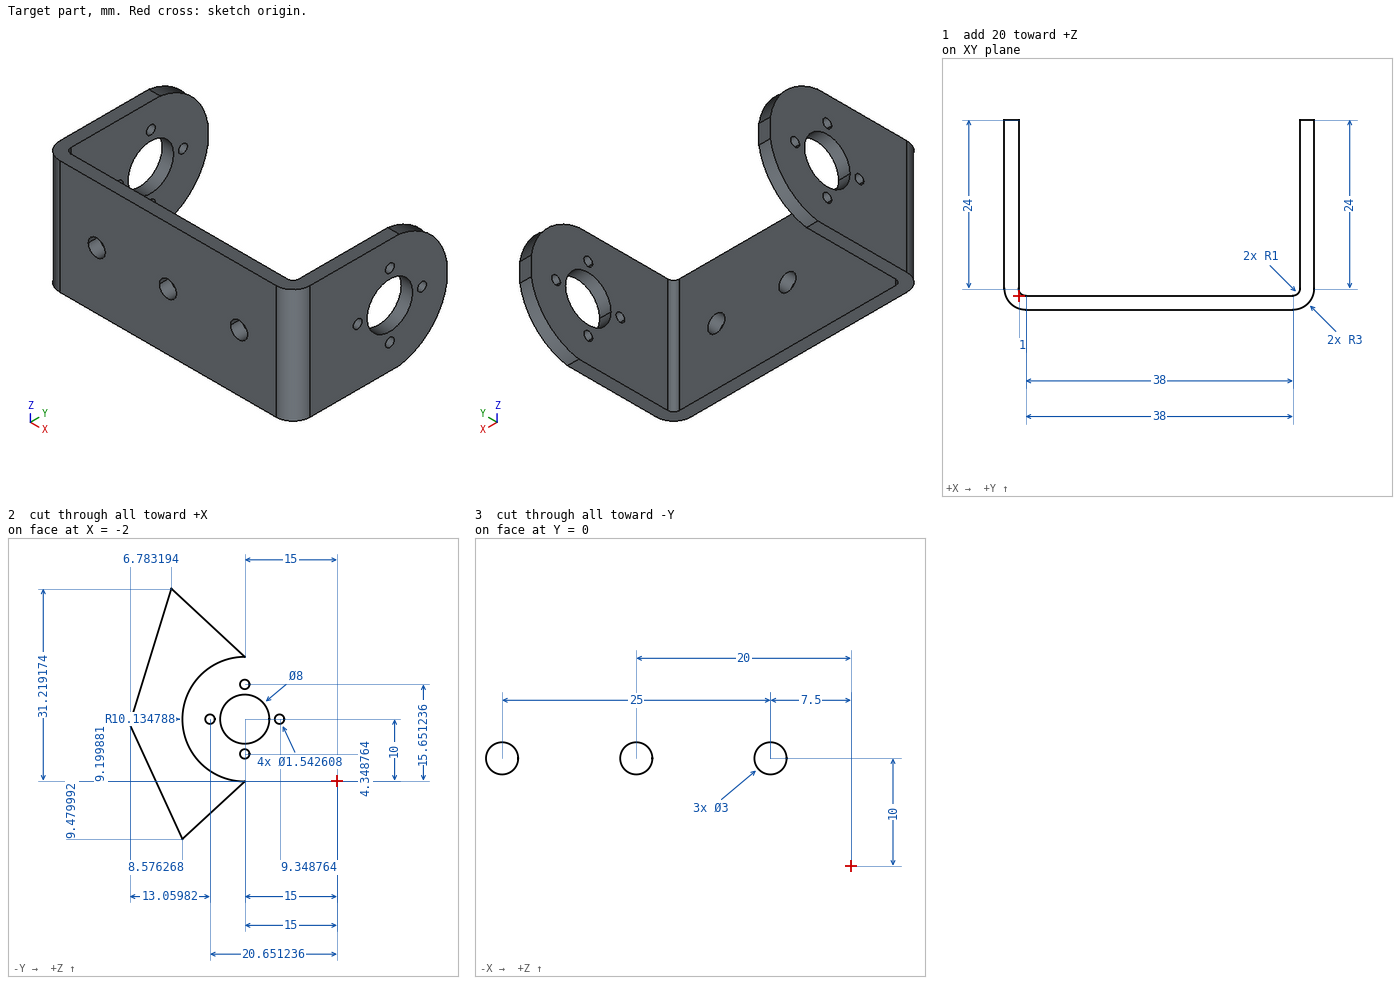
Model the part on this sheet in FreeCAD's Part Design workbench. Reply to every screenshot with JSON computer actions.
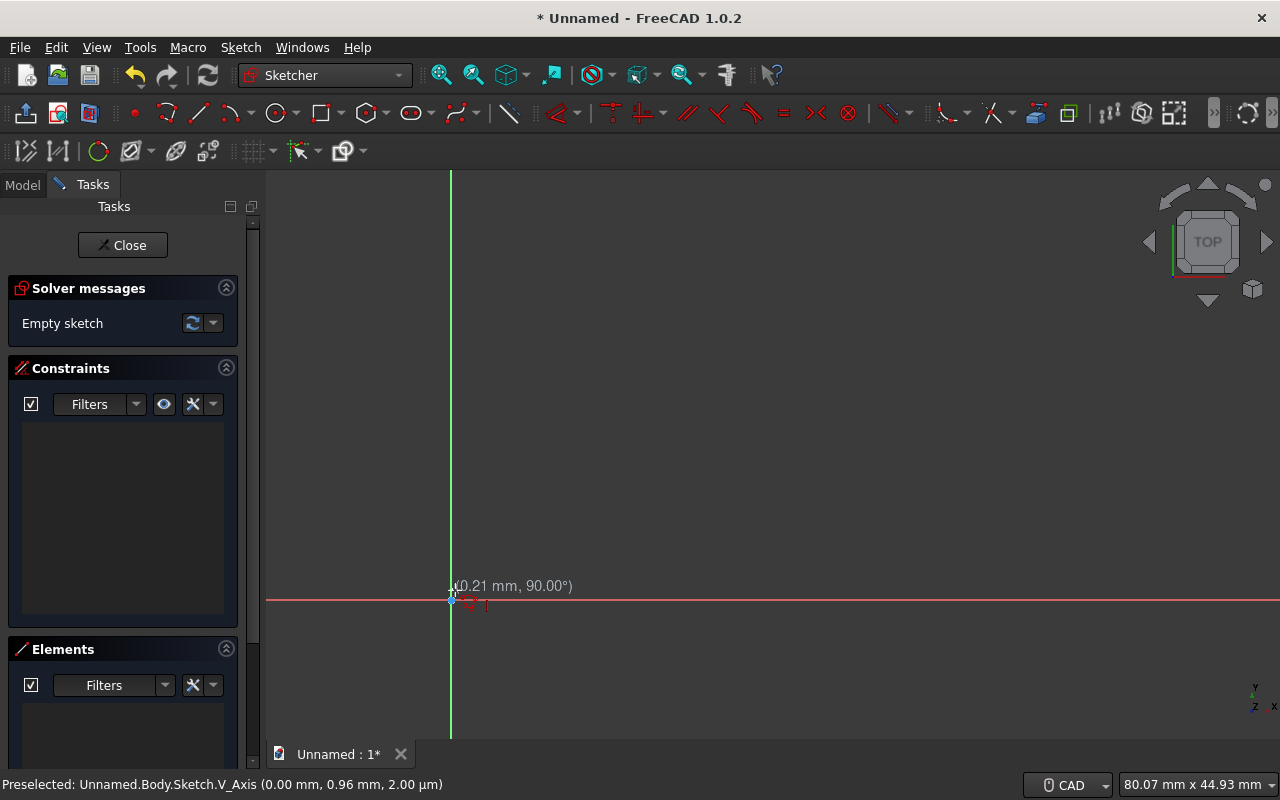
{"action": "left_click", "coordinate": [460, 284]}
{"action": "left_click", "coordinate": [426, 284]}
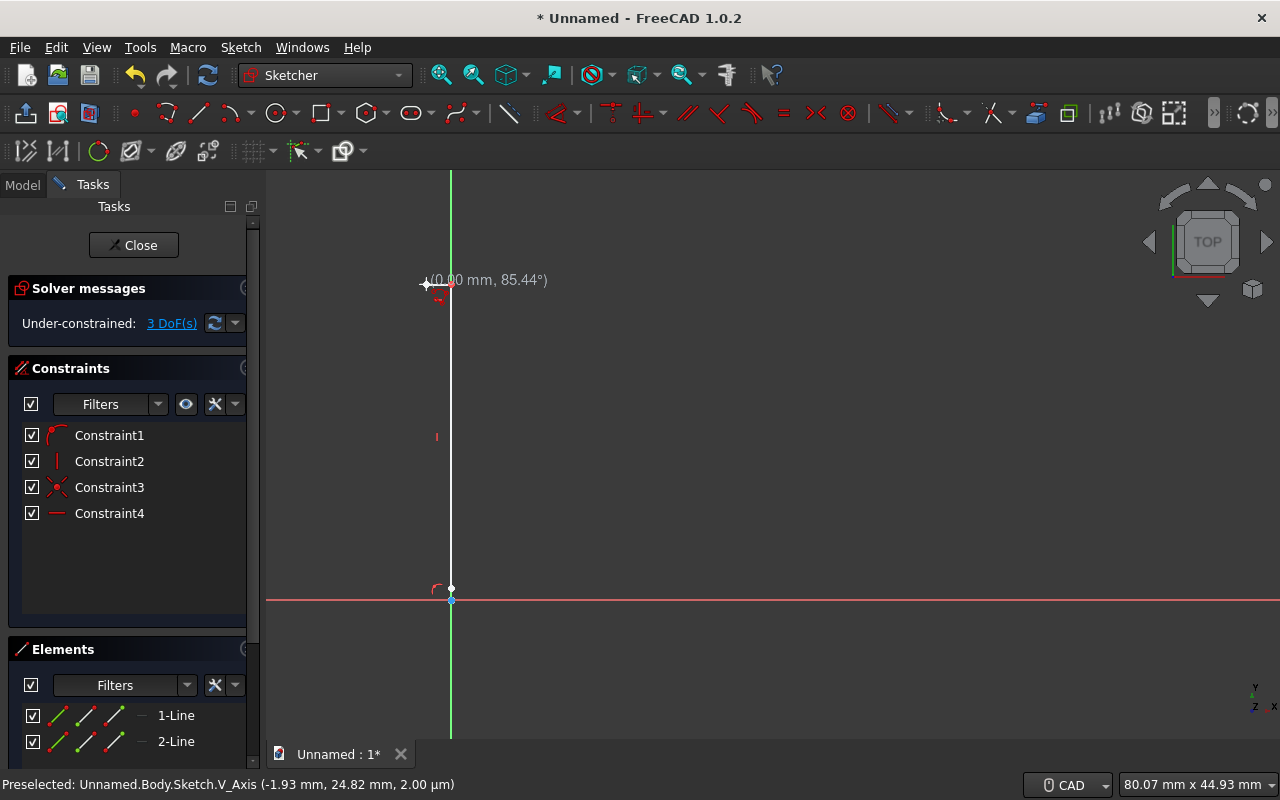
{"action": "scroll", "coordinate": [426, 588], "scroll_direction": "up", "scroll_amount": 2}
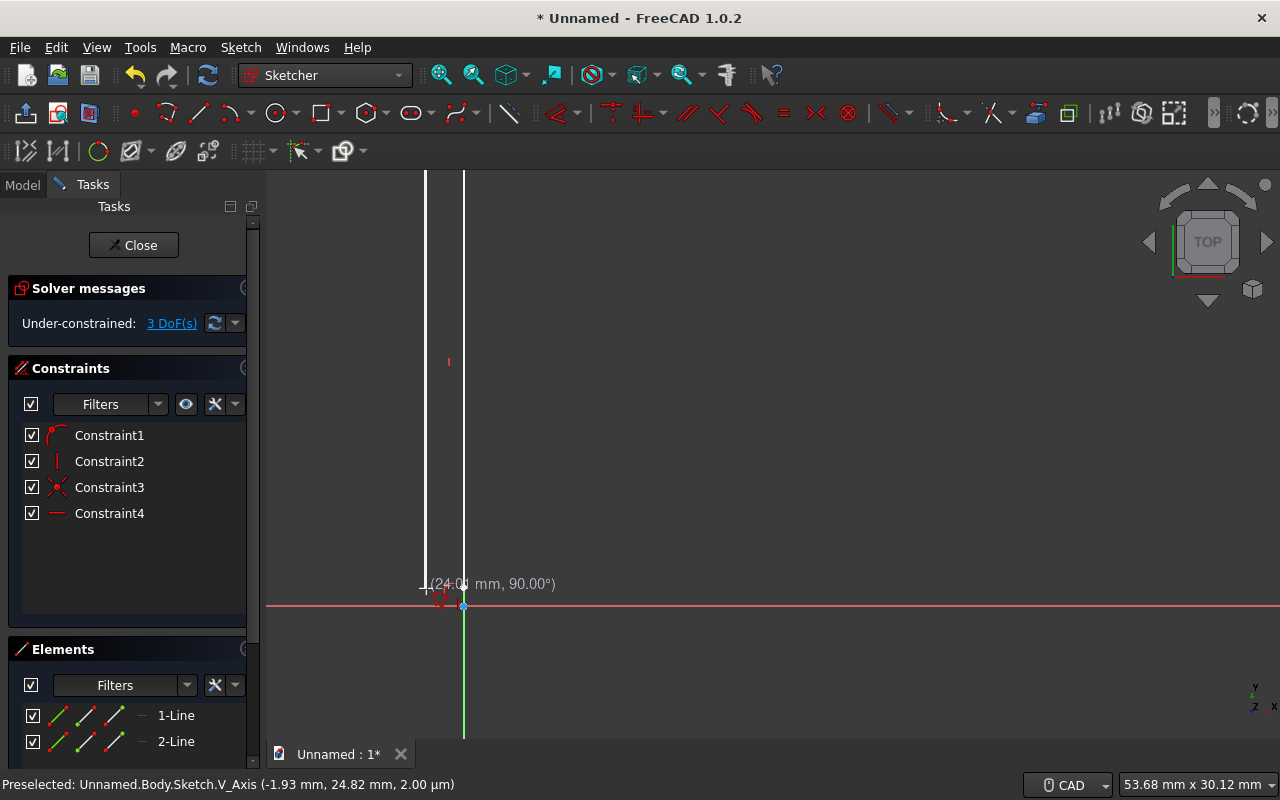
{"action": "left_click", "coordinate": [426, 587]}
{"action": "right_click", "coordinate": [426, 587]}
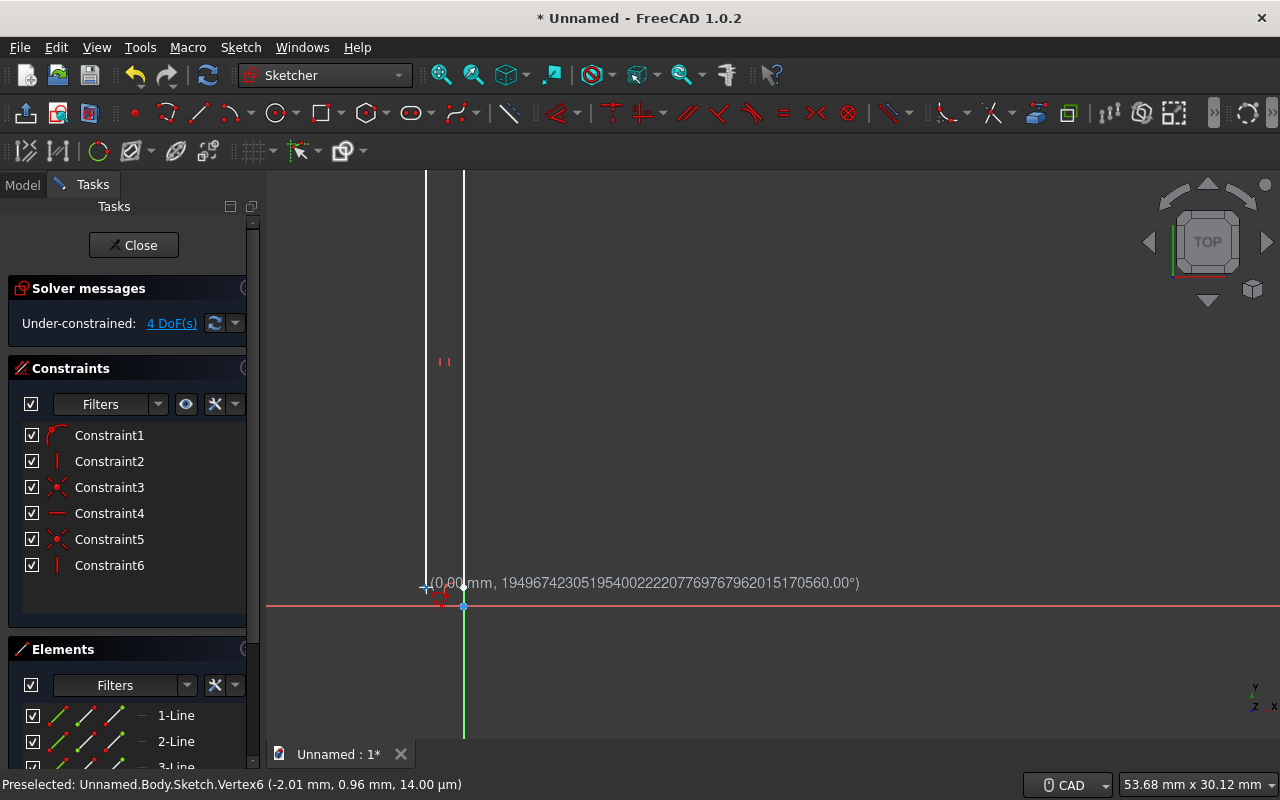
{"action": "left_click", "coordinate": [200, 114]}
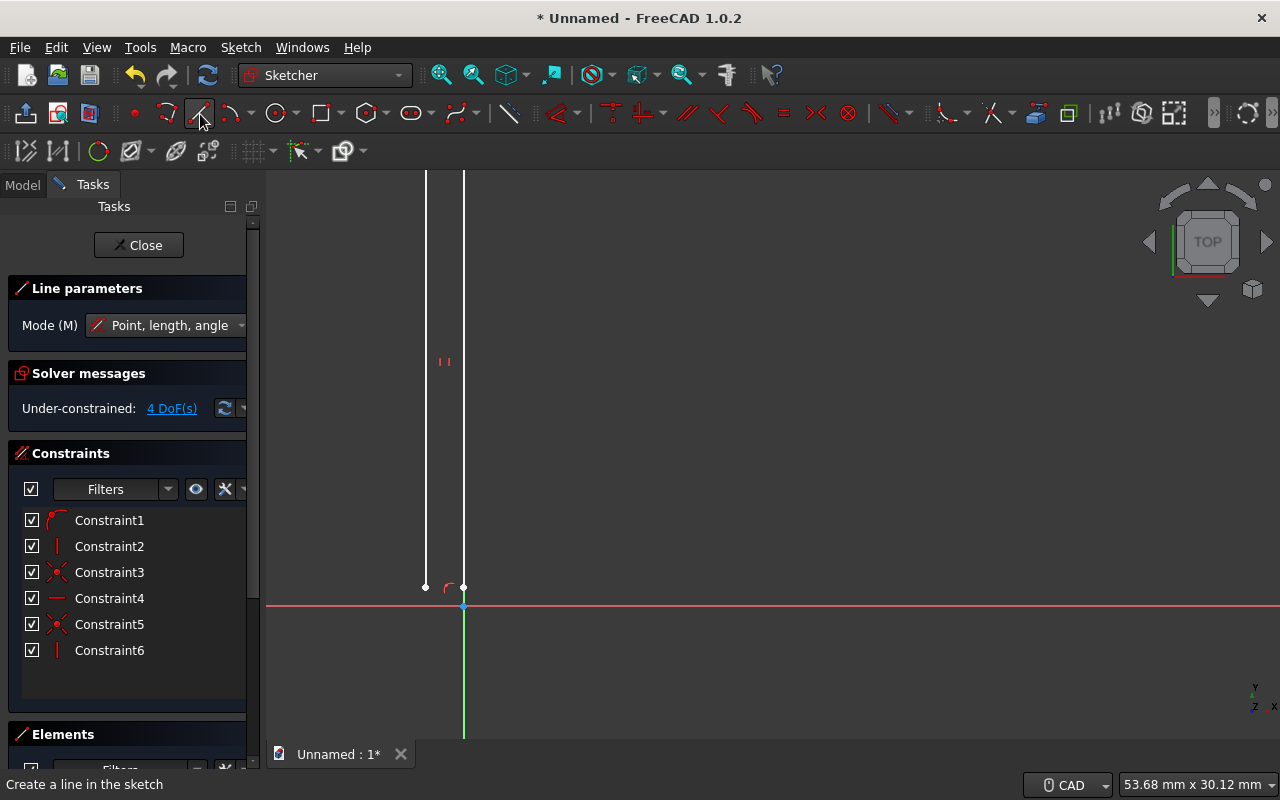
{"action": "left_click", "coordinate": [483, 644]}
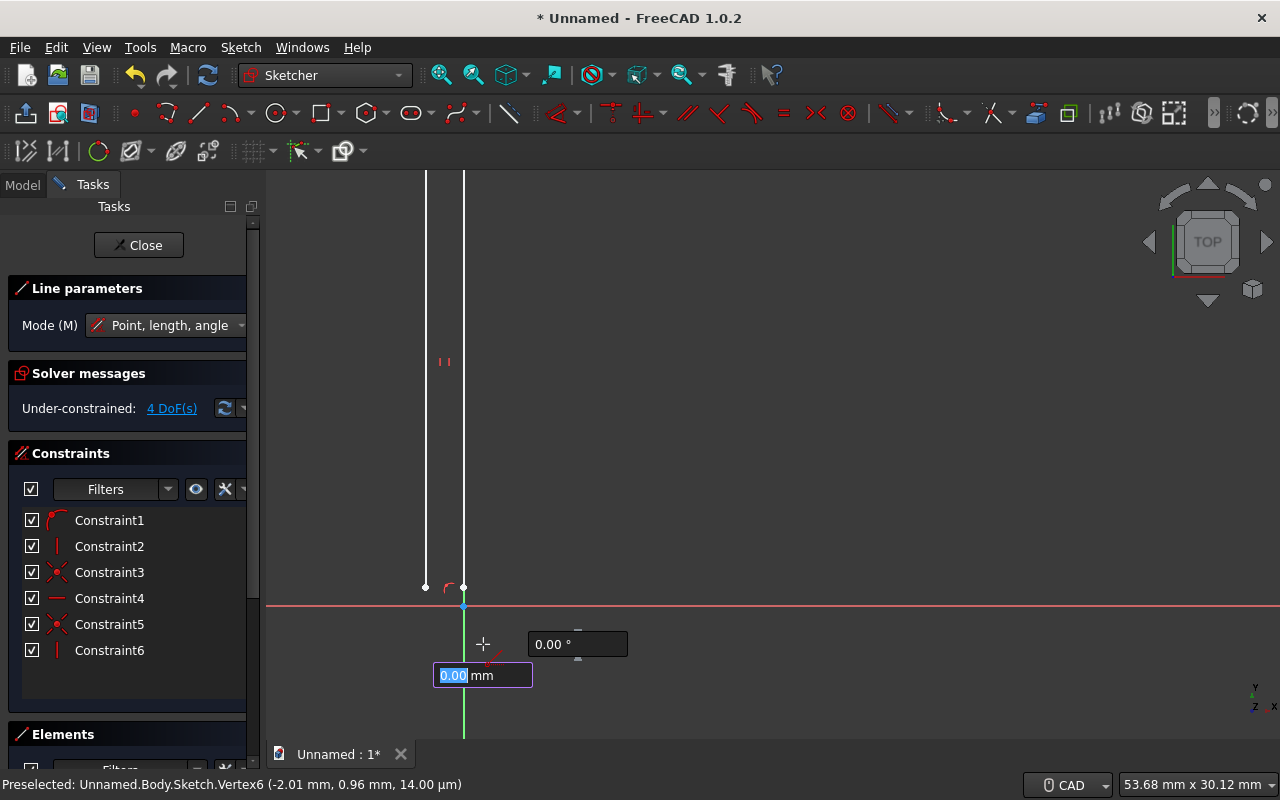
{"action": "scroll", "coordinate": [426, 588], "scroll_direction": "down", "scroll_amount": 2}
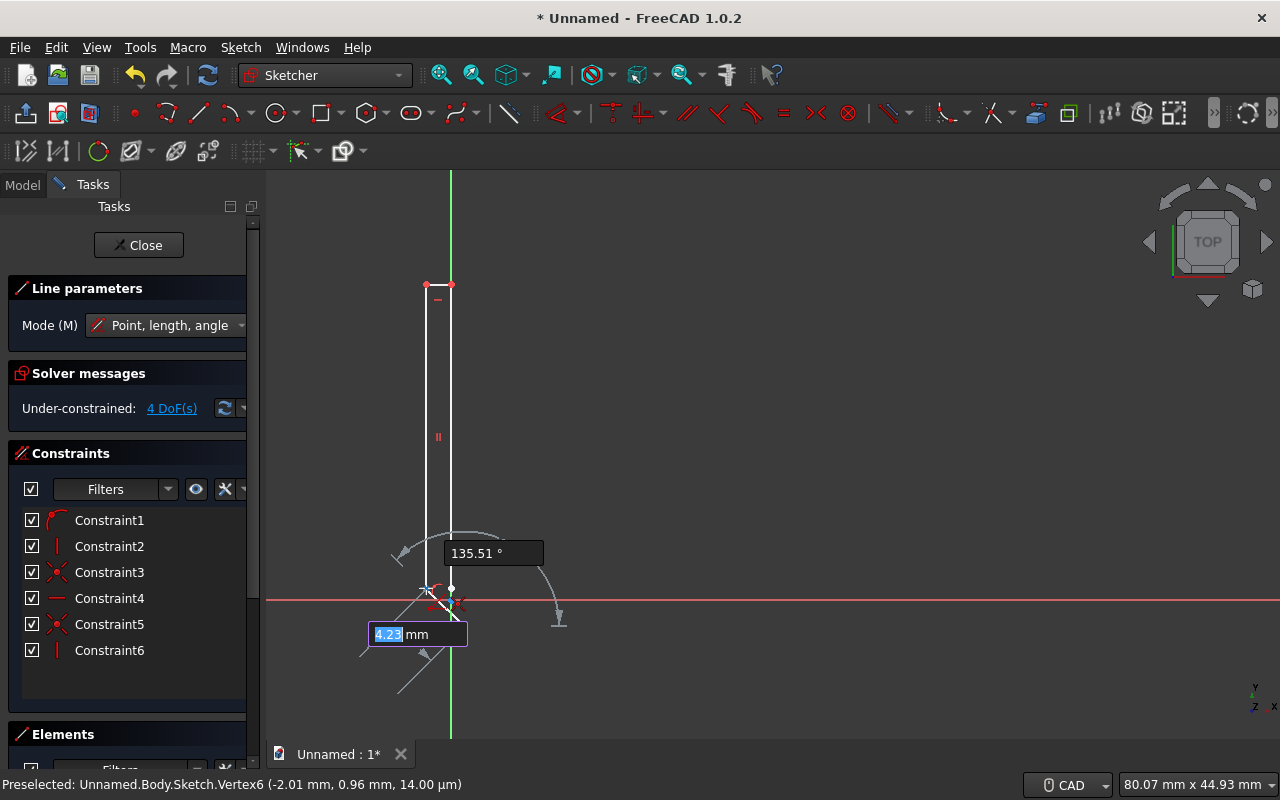
{"action": "left_click", "coordinate": [945, 626]}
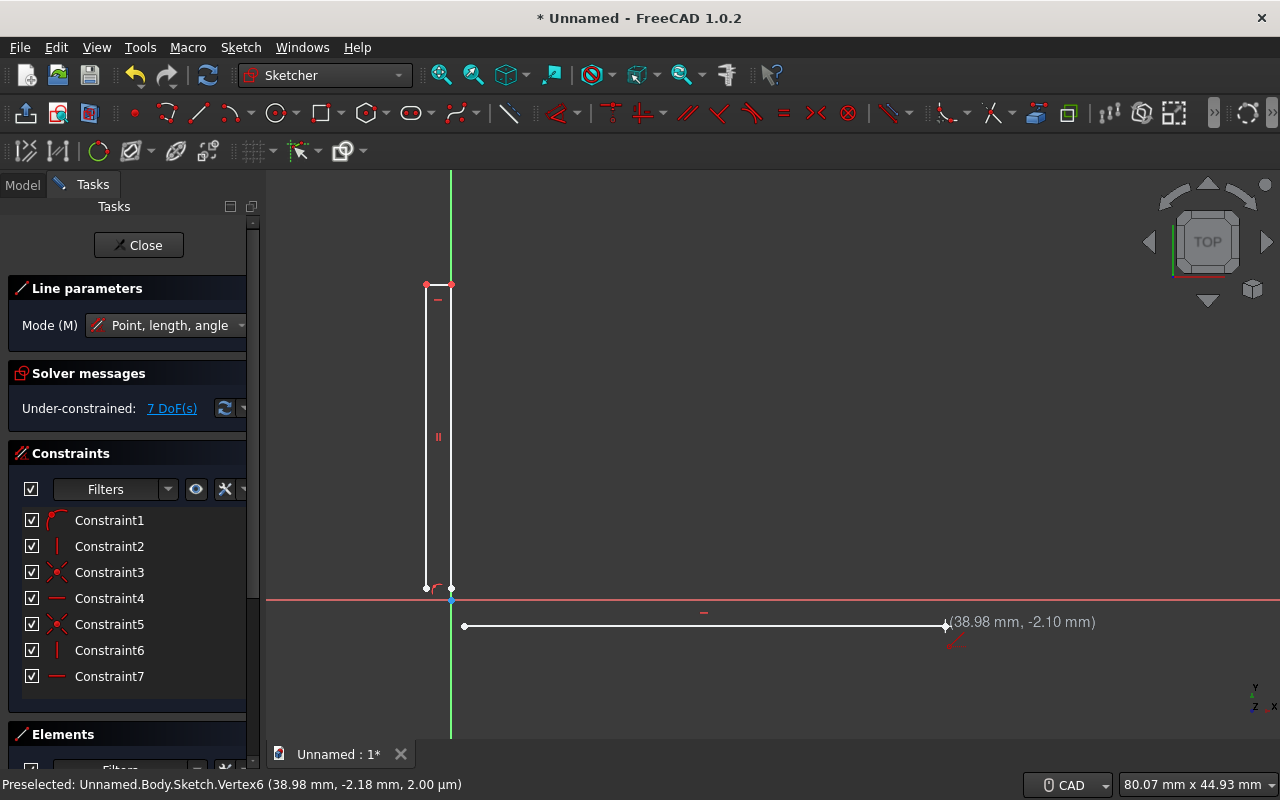
{"action": "left_click", "coordinate": [168, 114]}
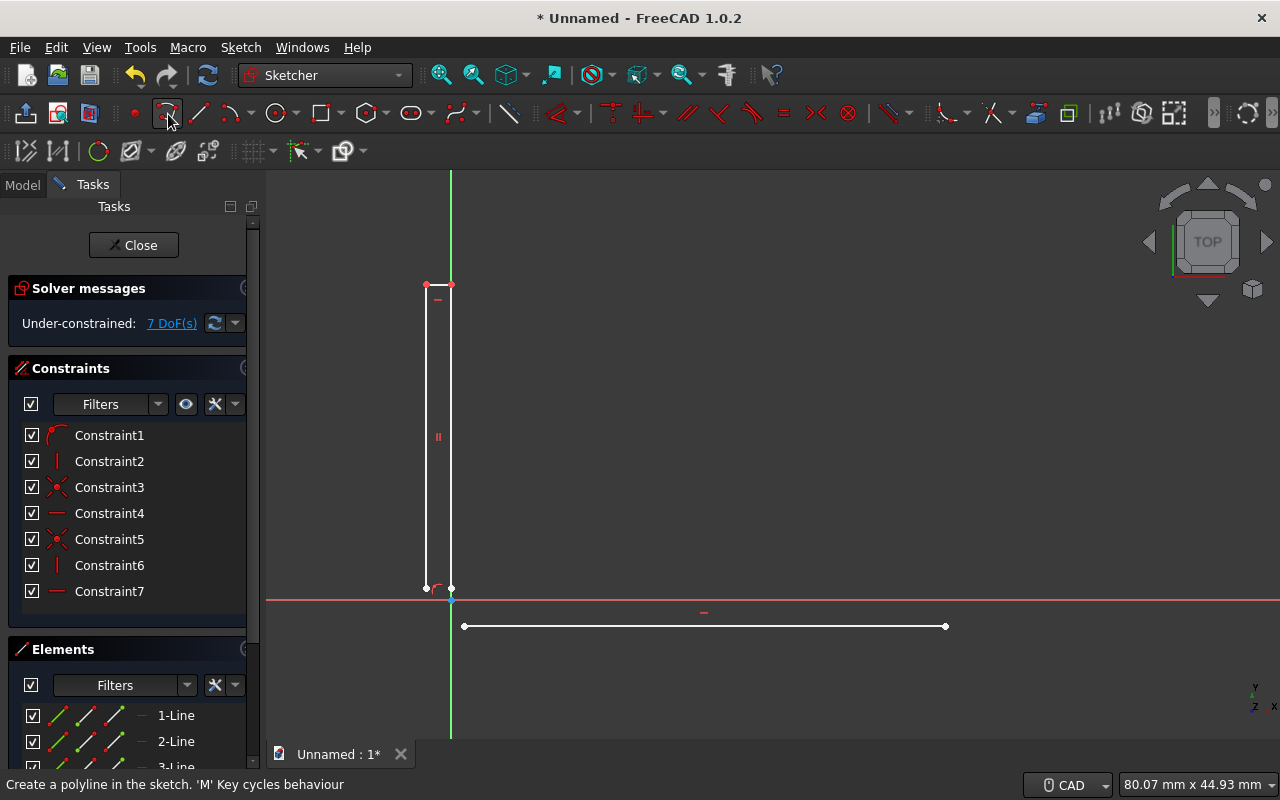
{"action": "scroll", "coordinate": [983, 588], "scroll_direction": "up", "scroll_amount": 2}